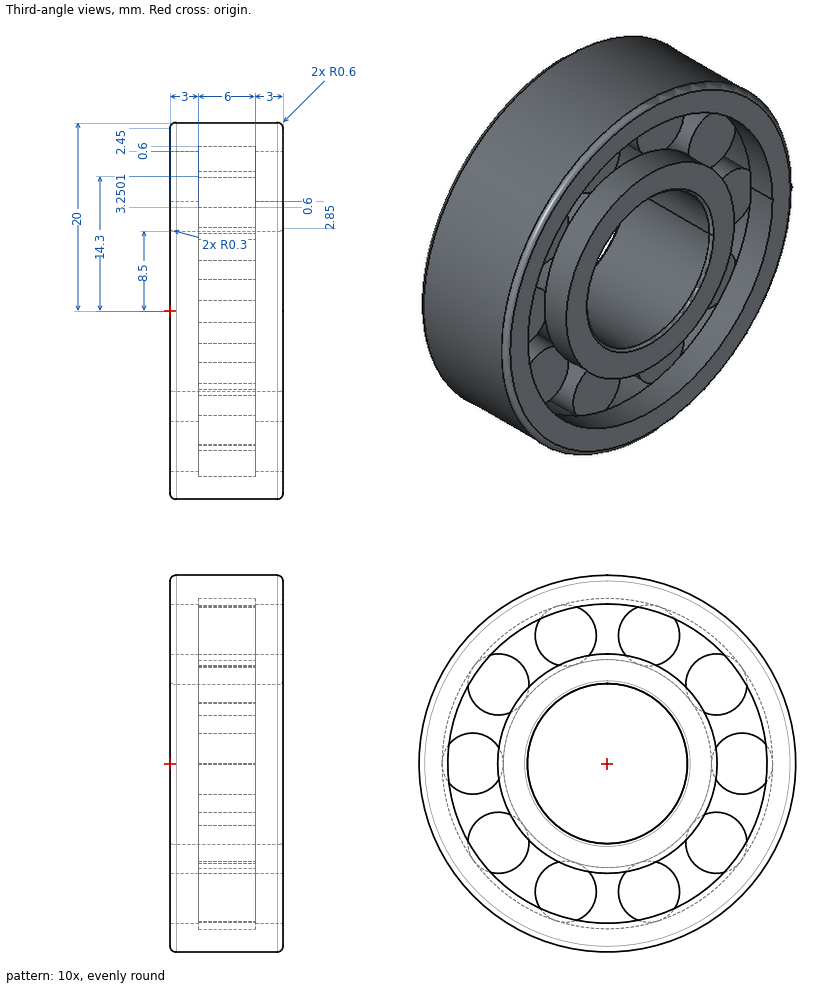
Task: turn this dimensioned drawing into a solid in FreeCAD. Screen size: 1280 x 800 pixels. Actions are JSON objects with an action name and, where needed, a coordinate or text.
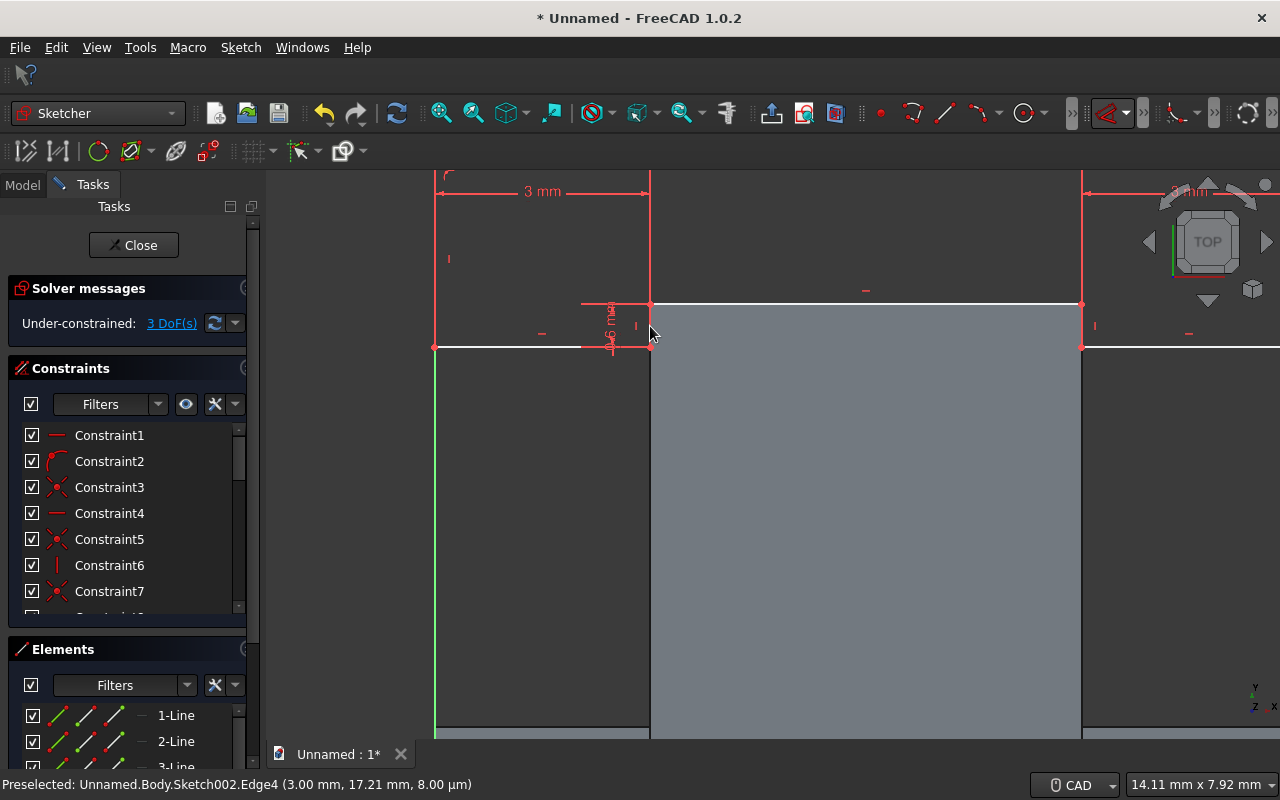
{"action": "left_click", "coordinate": [1082, 317]}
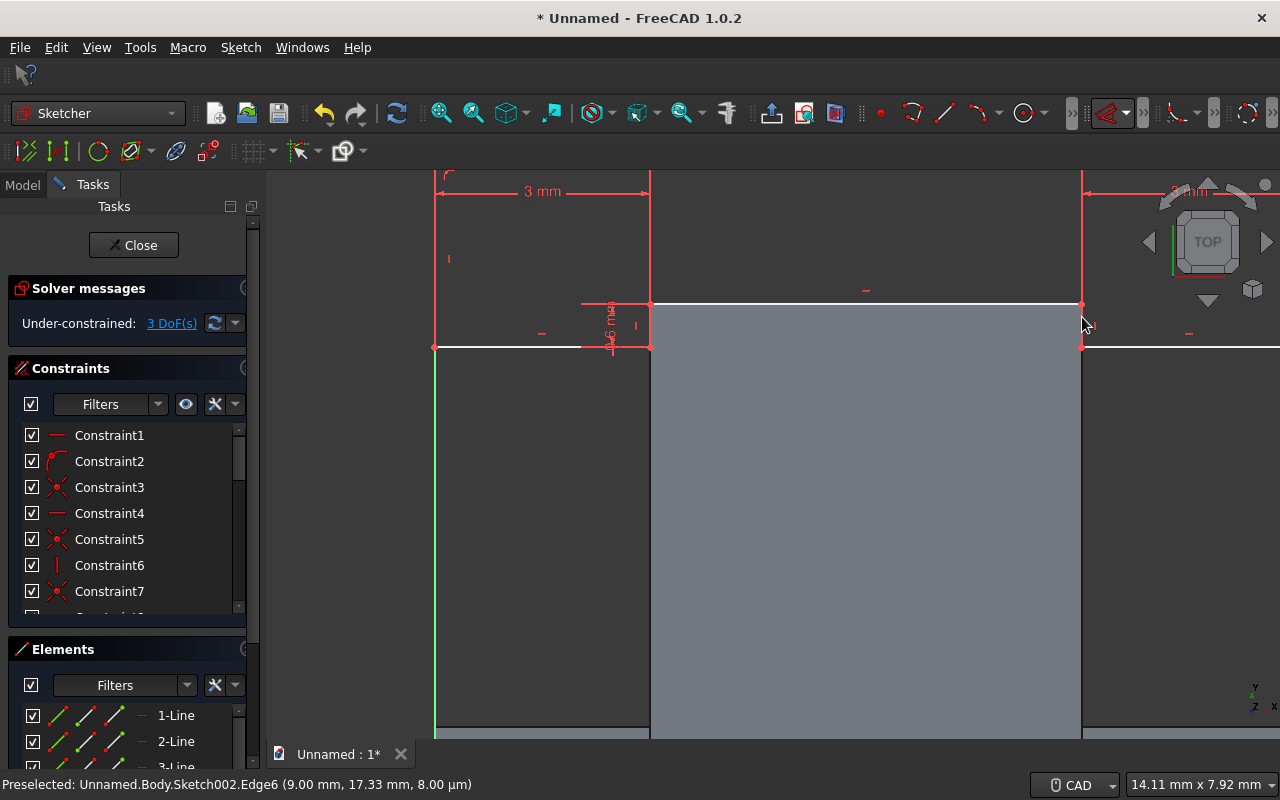
{"action": "left_click", "coordinate": [1128, 114]}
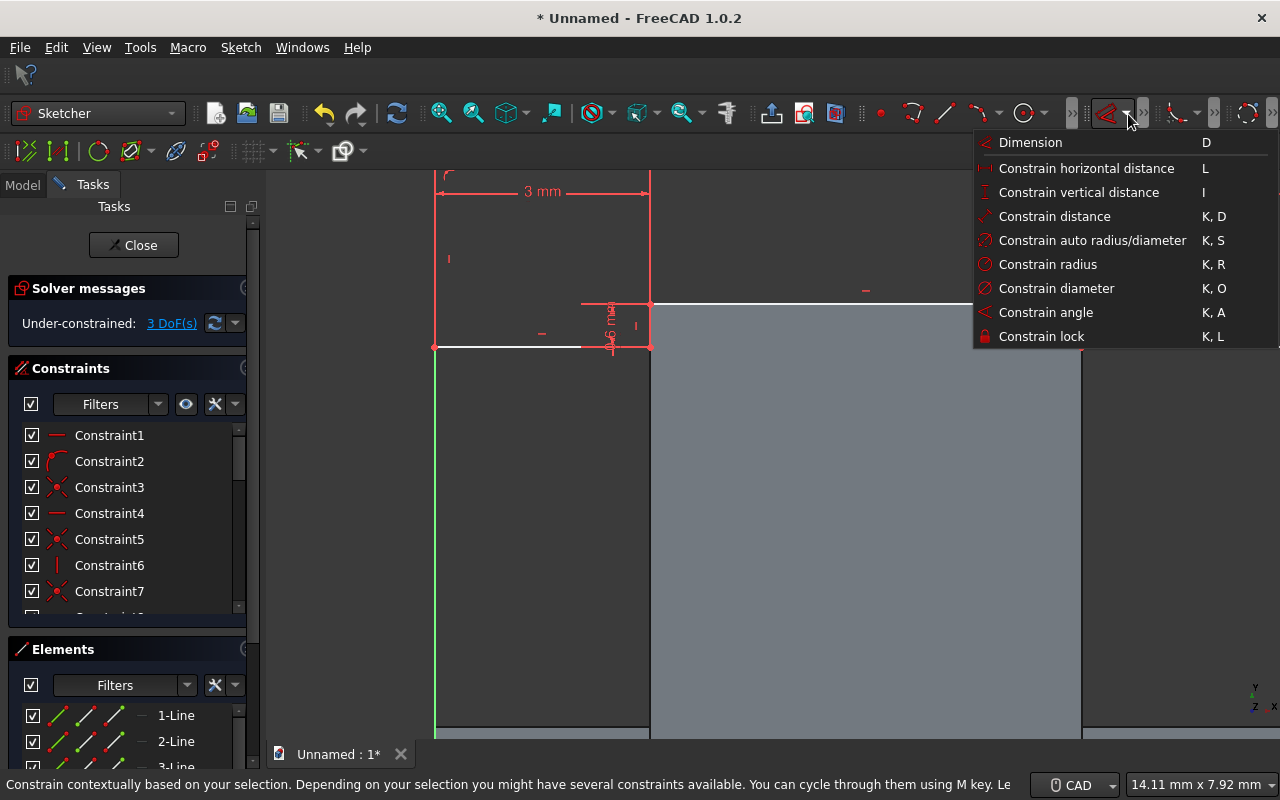
{"action": "left_click", "coordinate": [1126, 192]}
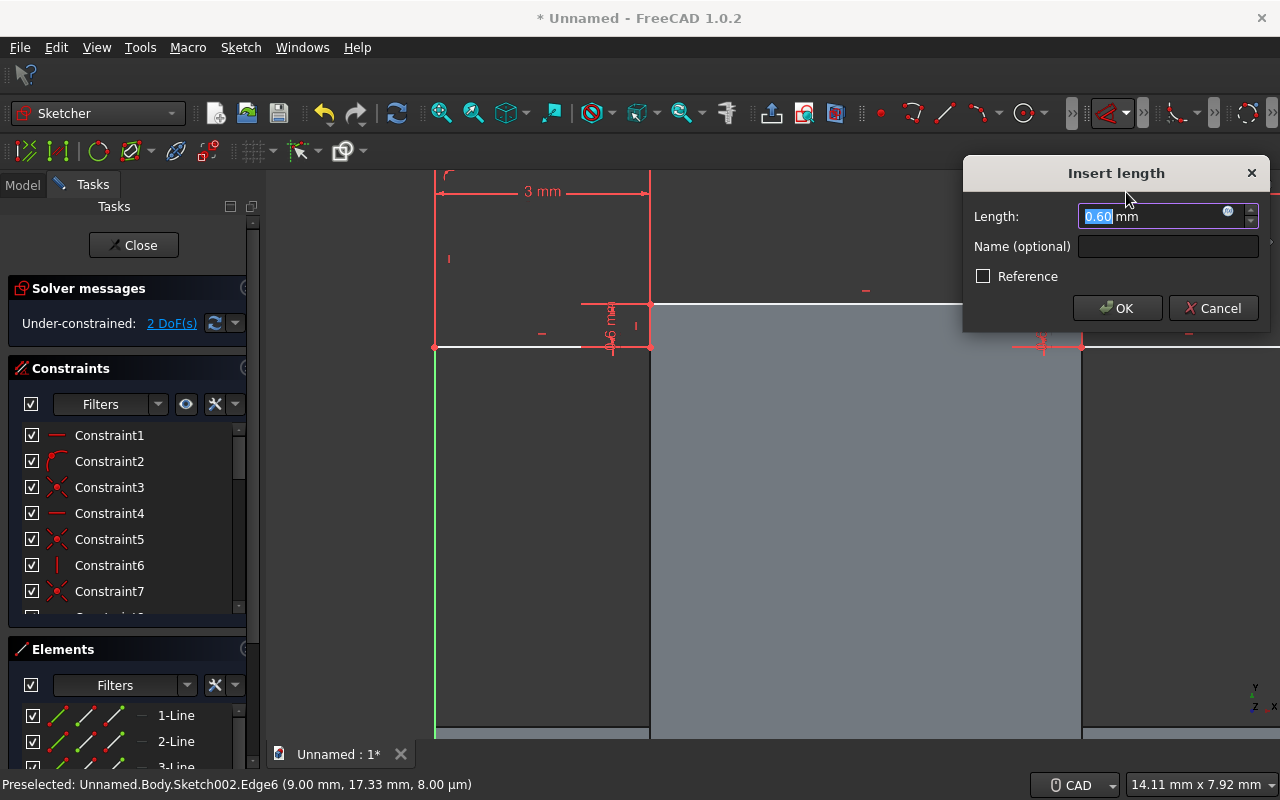
{"action": "type", "text": "0.6"}
{"action": "key", "text": "Return"}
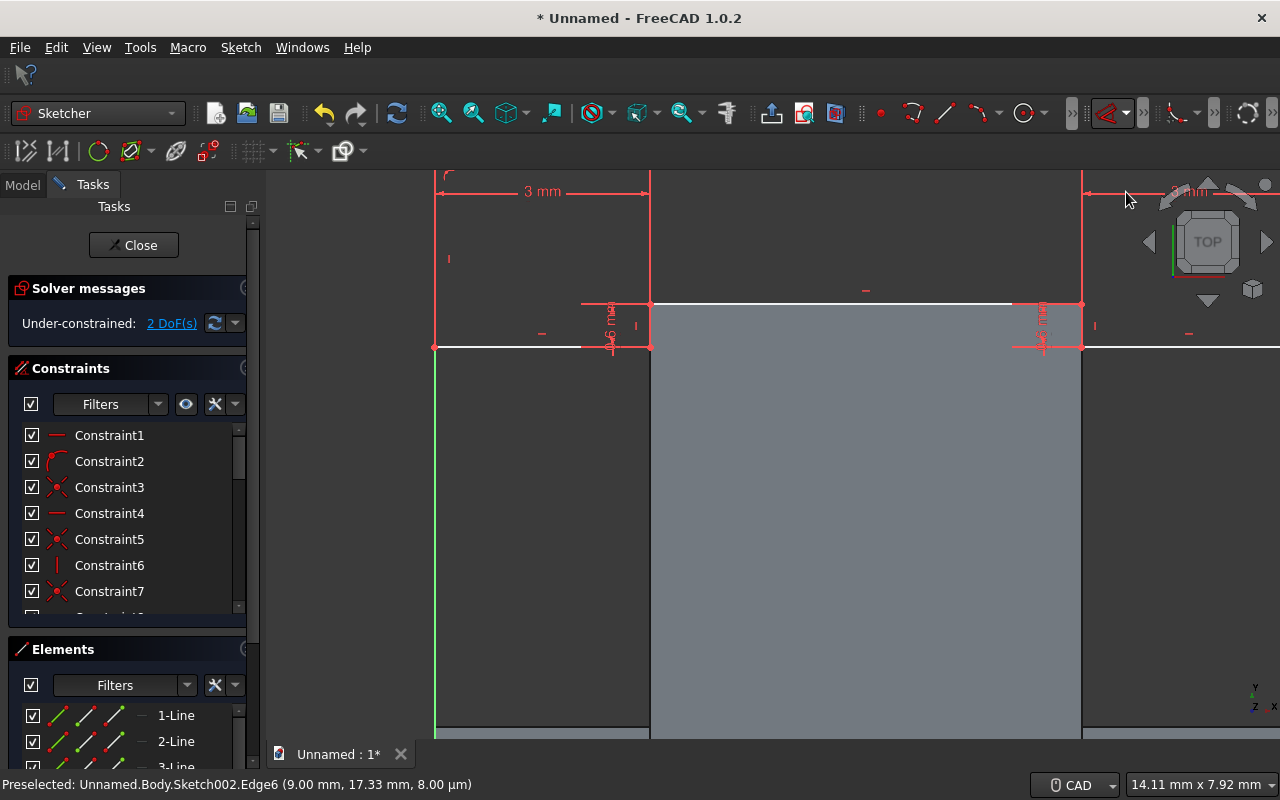
{"action": "scroll", "coordinate": [652, 327], "scroll_direction": "down", "scroll_amount": 7}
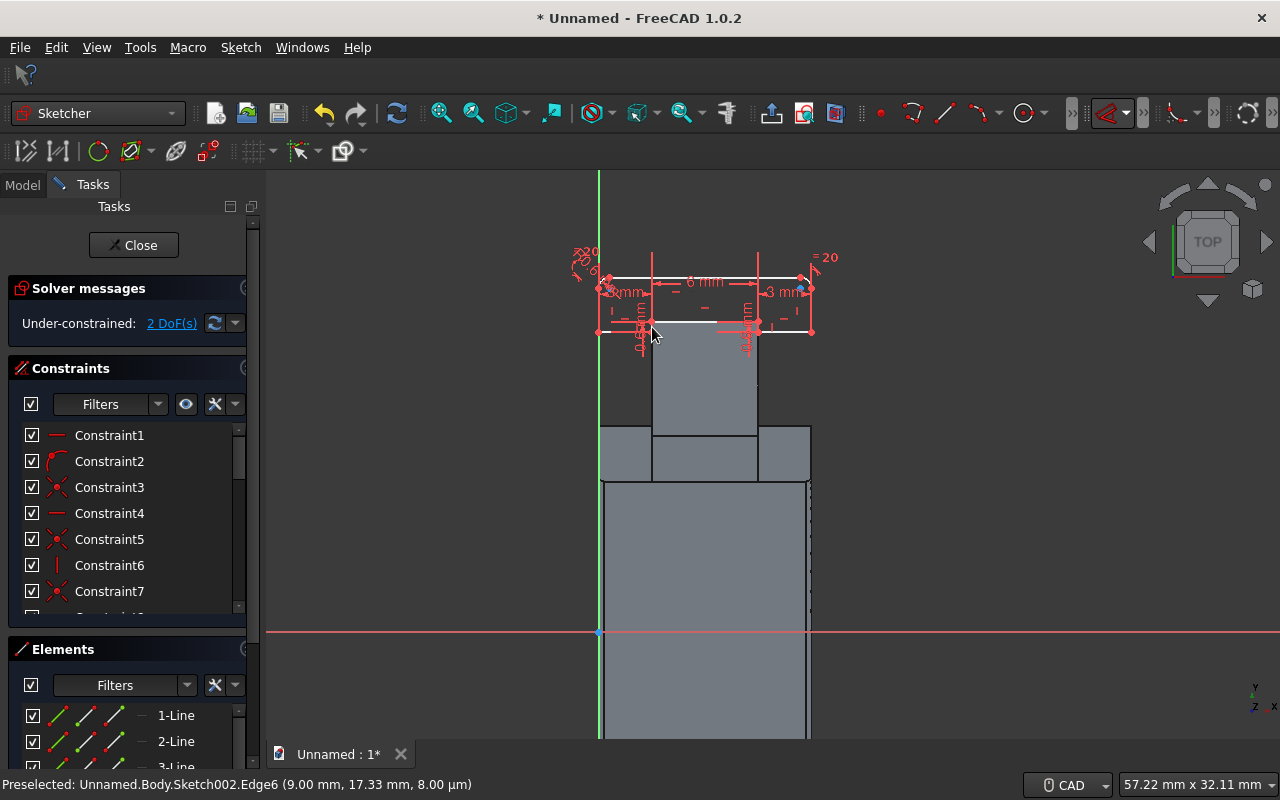
{"action": "left_click", "coordinate": [801, 278]}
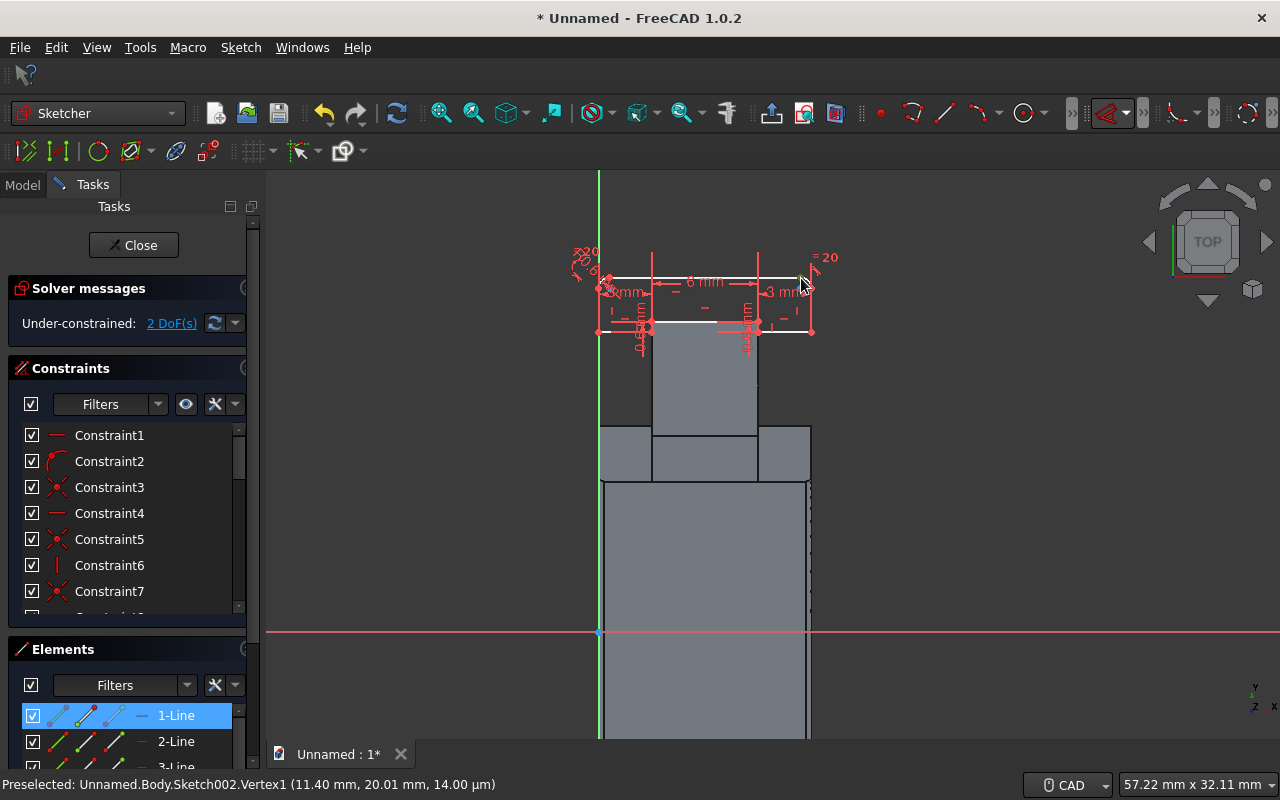
{"action": "key", "text": "i"}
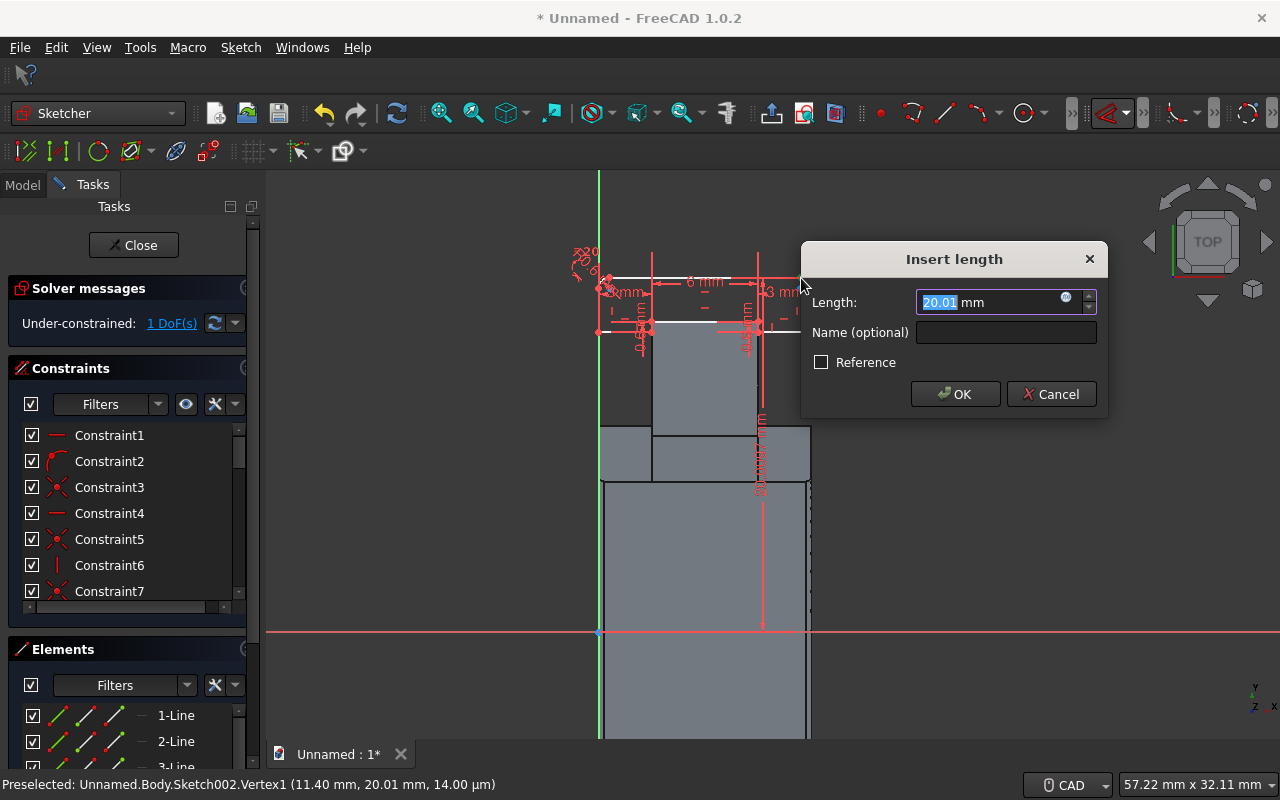
{"action": "type", "text": "20"}
{"action": "key", "text": "Return"}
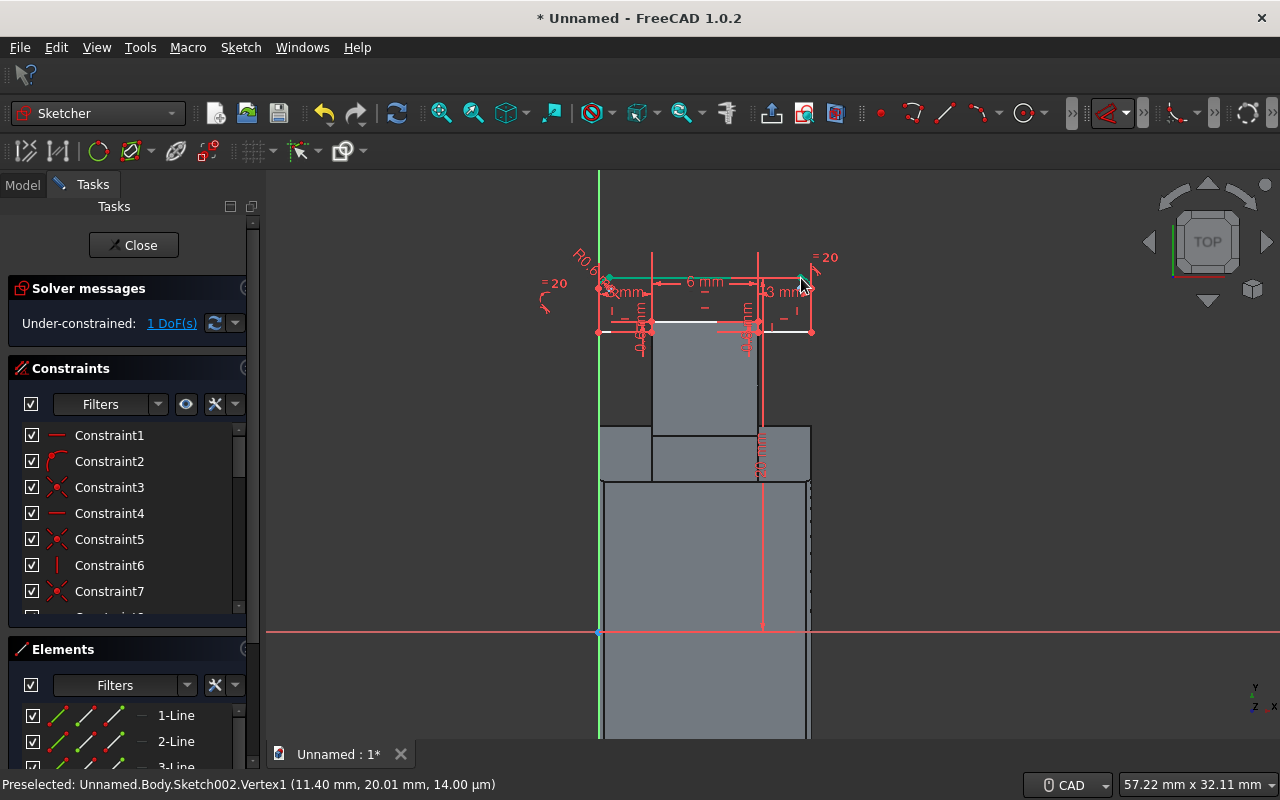
{"action": "left_click", "coordinate": [599, 302]}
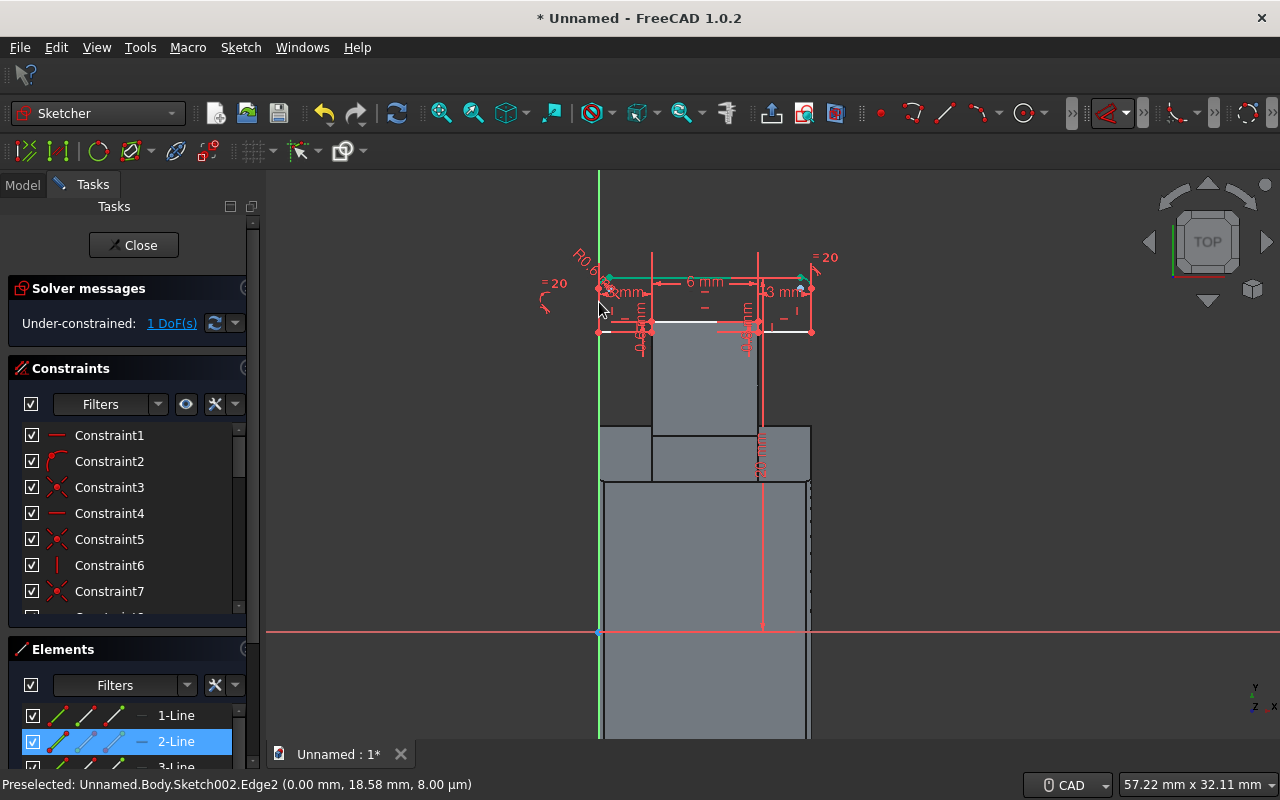
{"action": "left_click", "coordinate": [1128, 114]}